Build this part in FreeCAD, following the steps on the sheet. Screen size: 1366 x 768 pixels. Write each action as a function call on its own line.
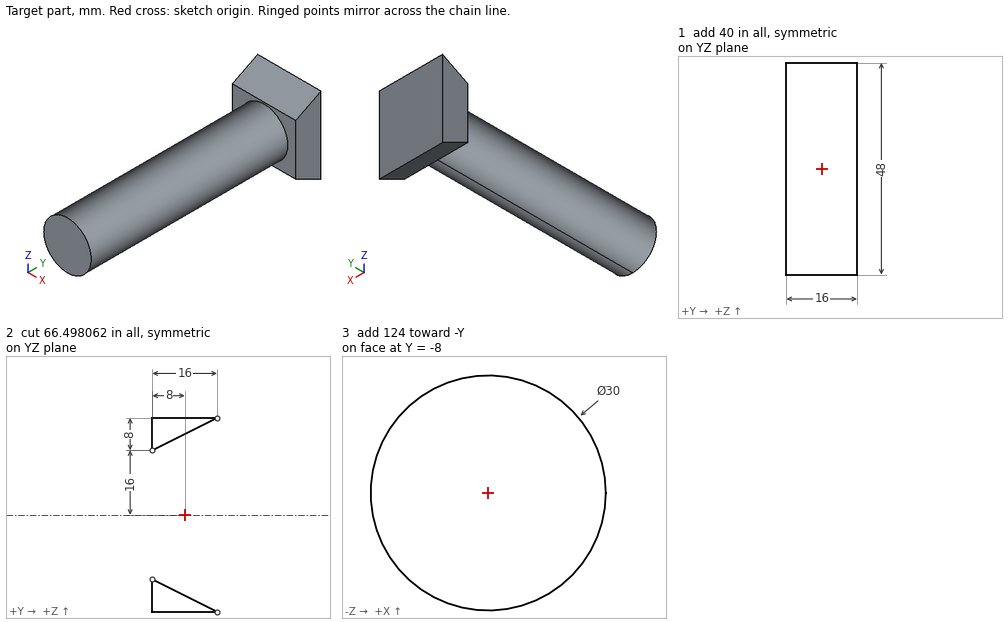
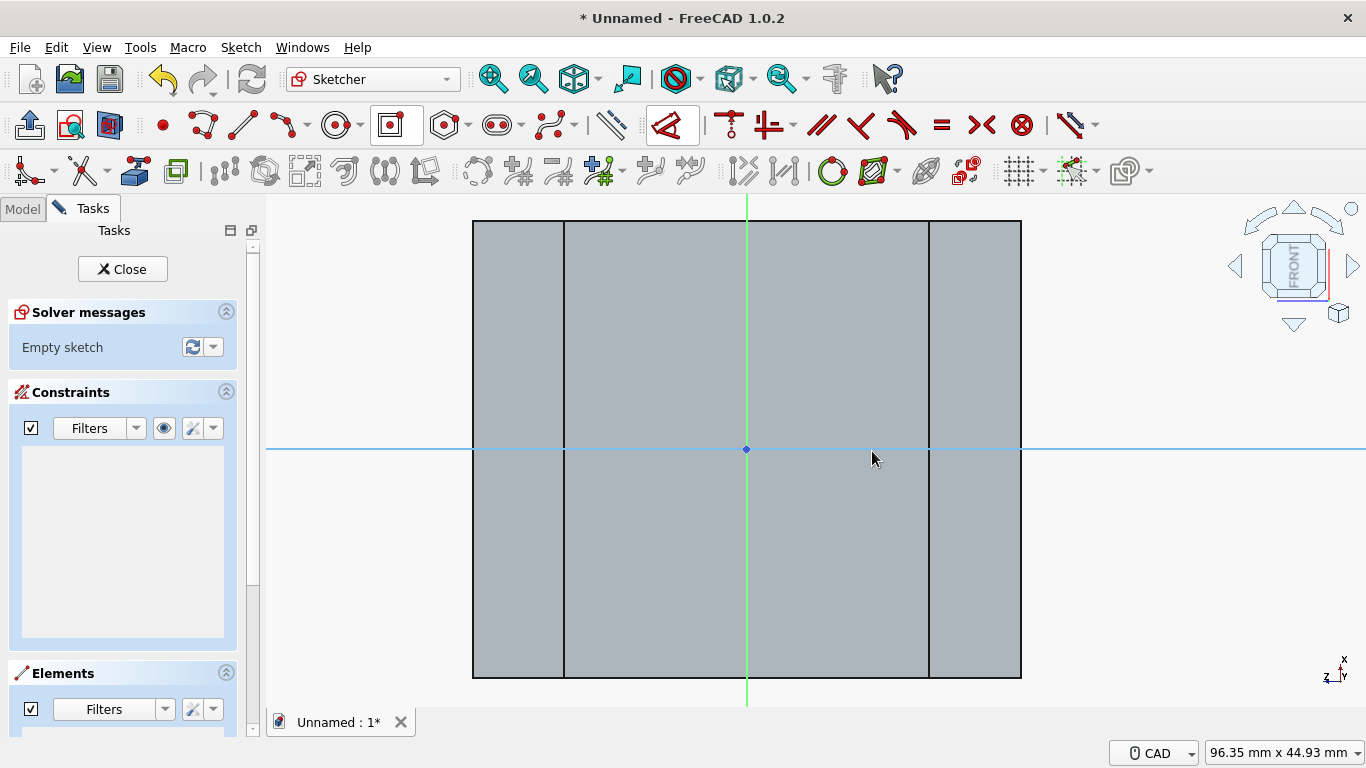
click(336, 126)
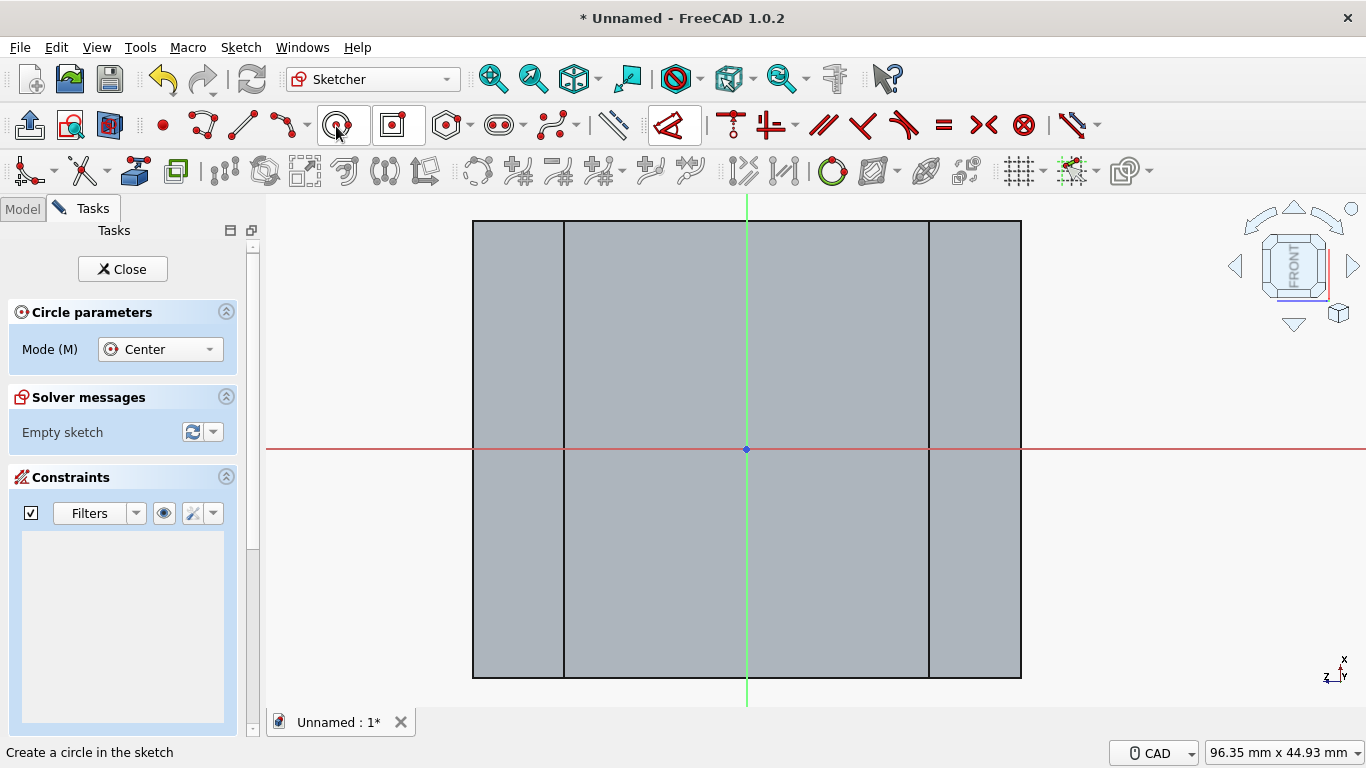
click(747, 449)
move(868, 328)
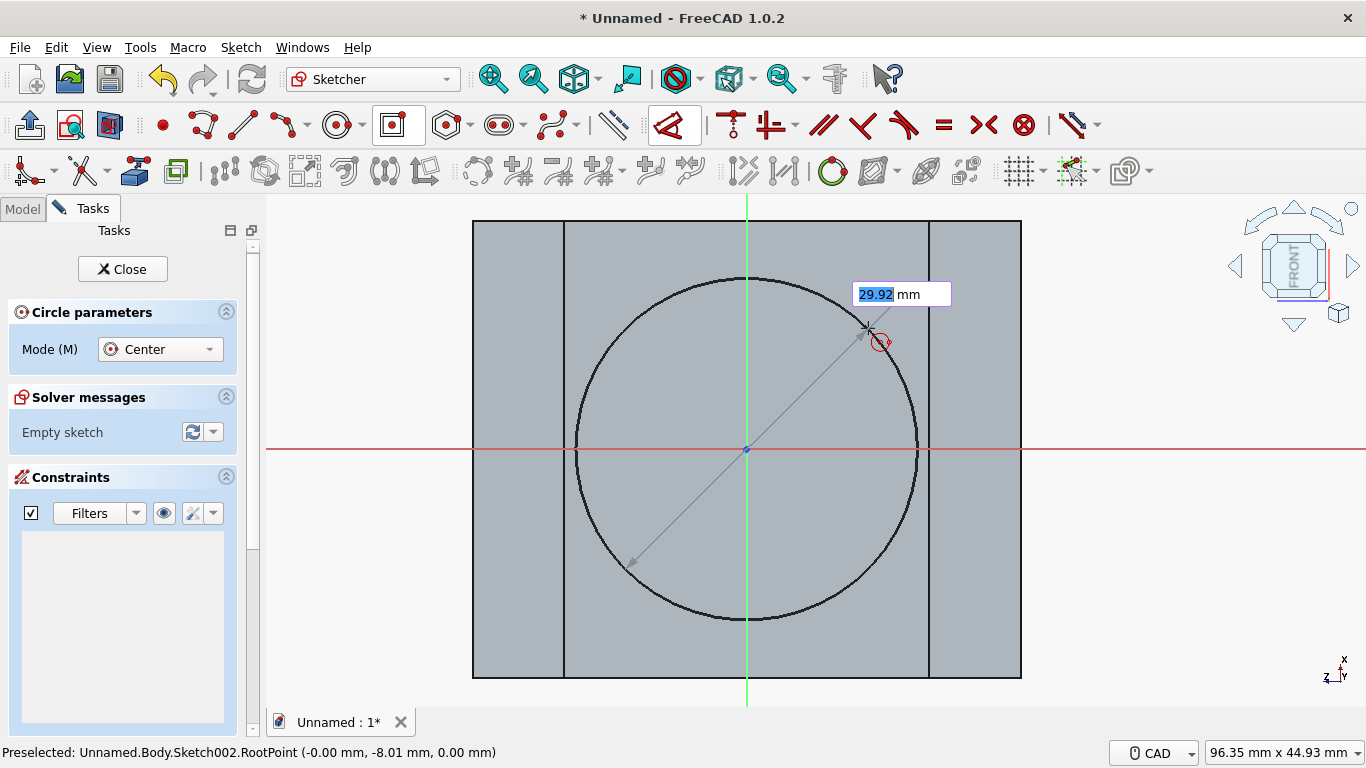
text(30)
key(Return)
key(Escape)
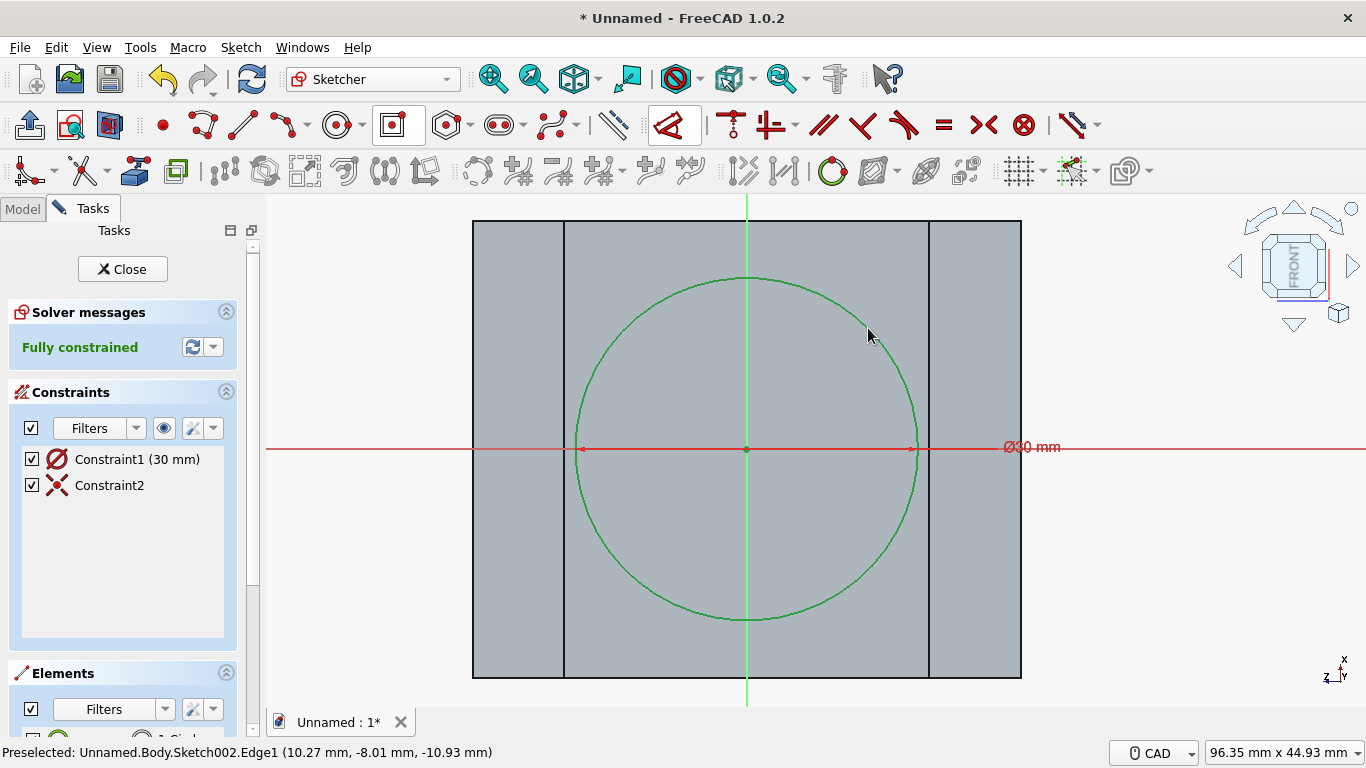
click(123, 269)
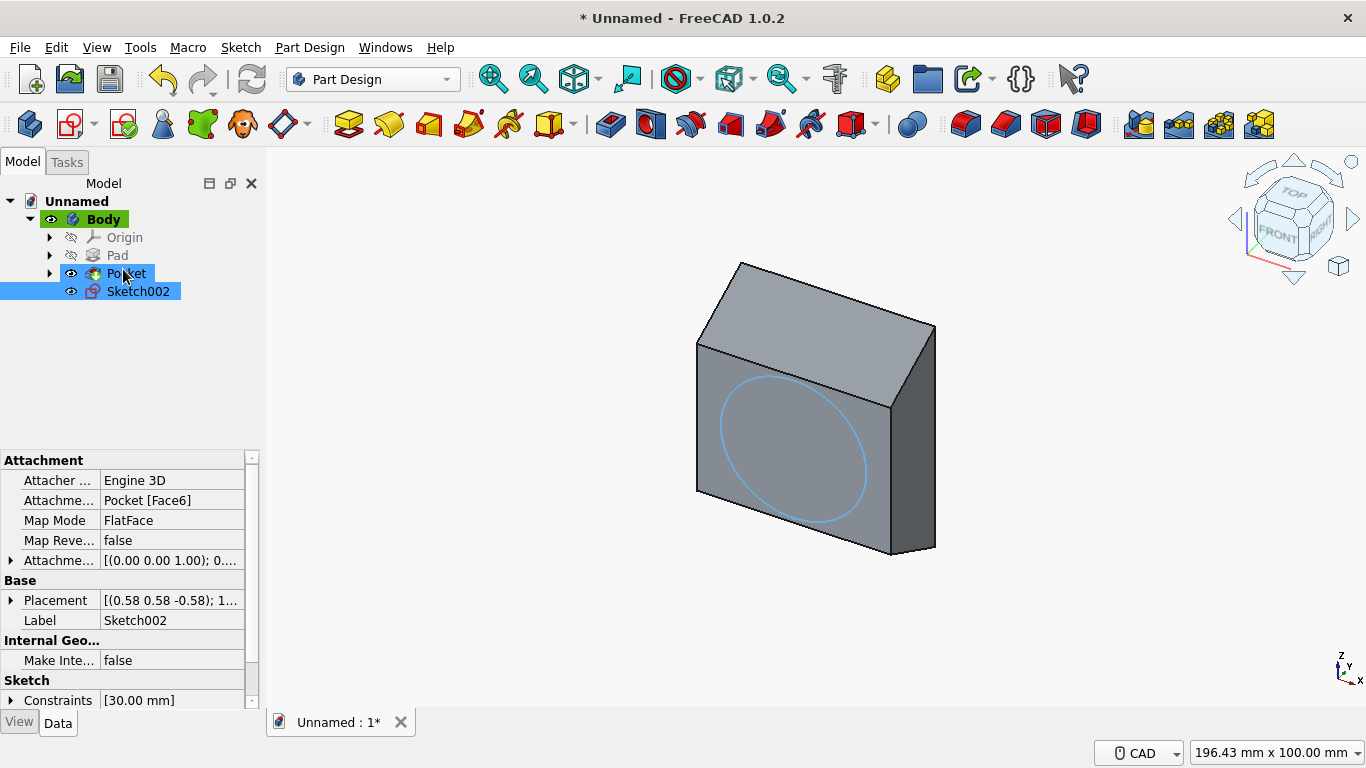
click(350, 124)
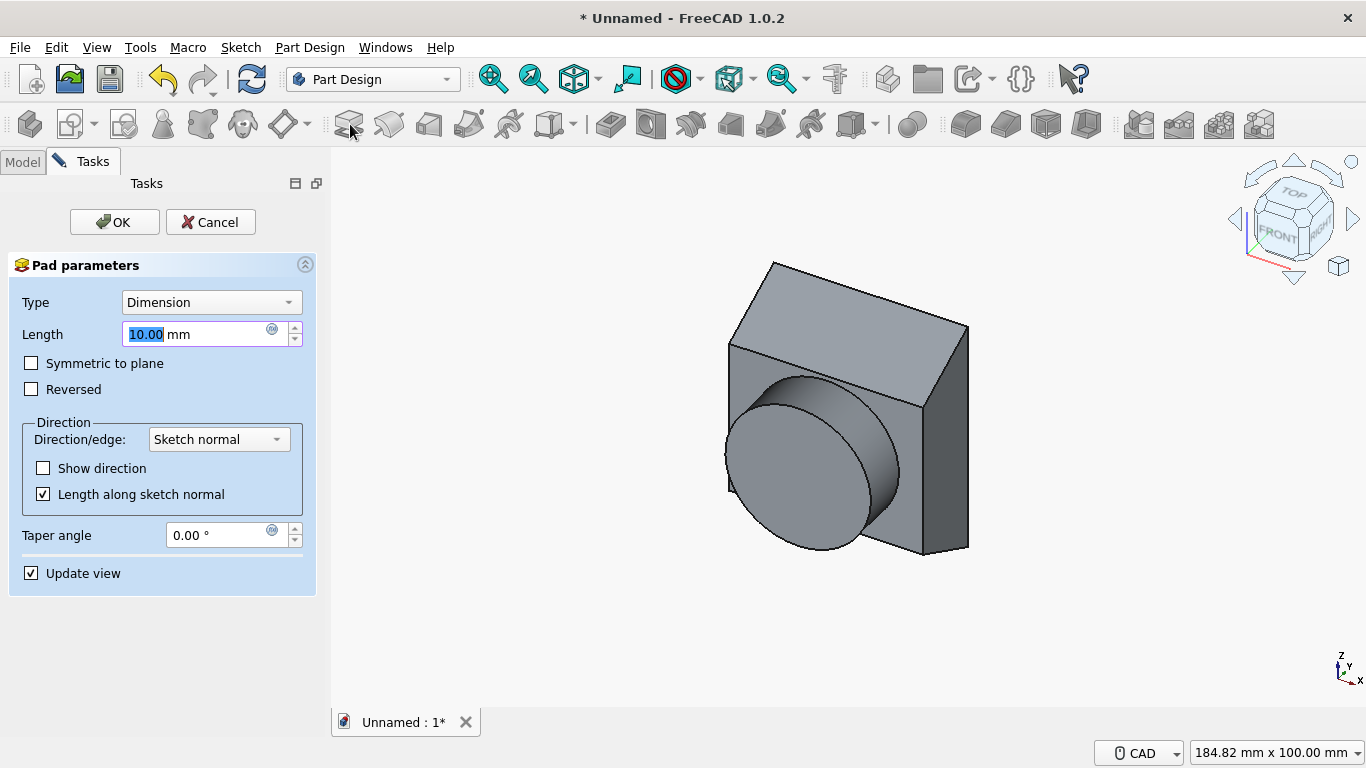
text(124)
key(Tab)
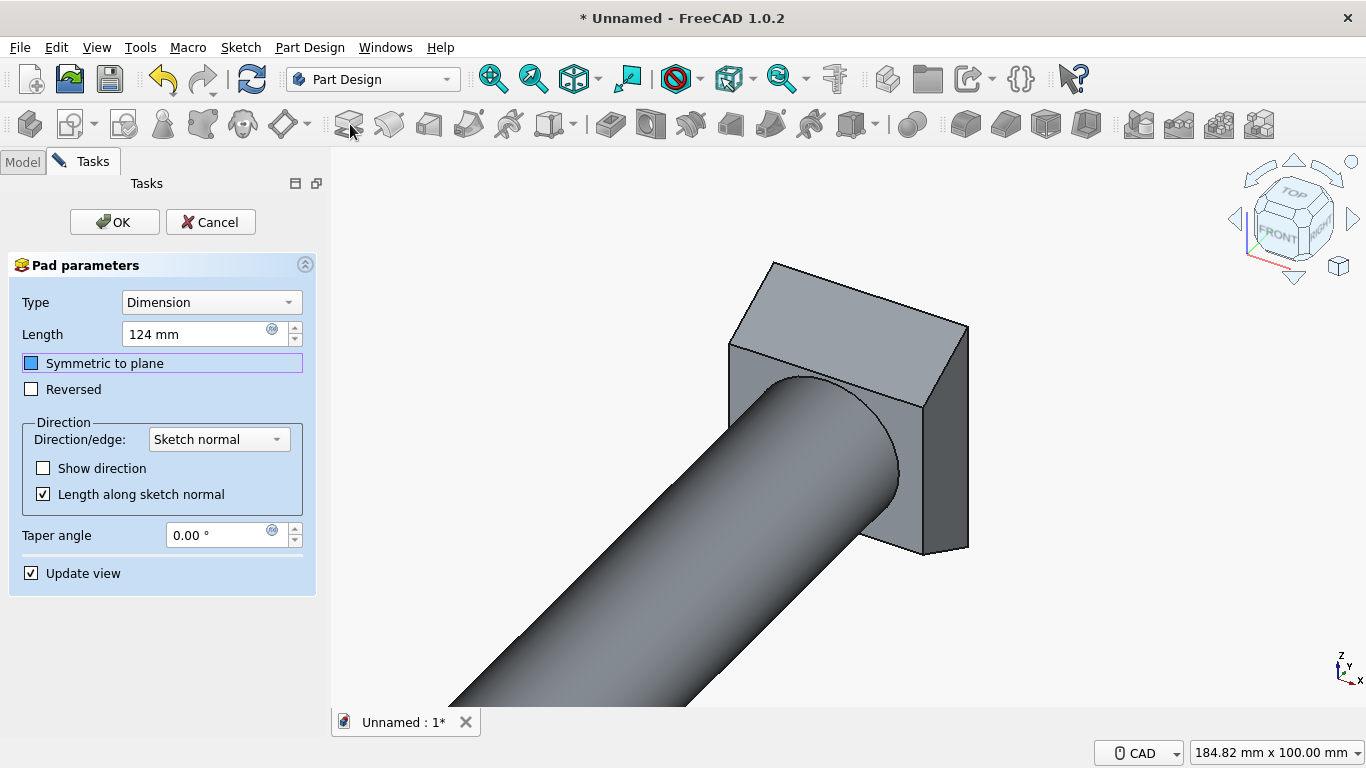
click(115, 222)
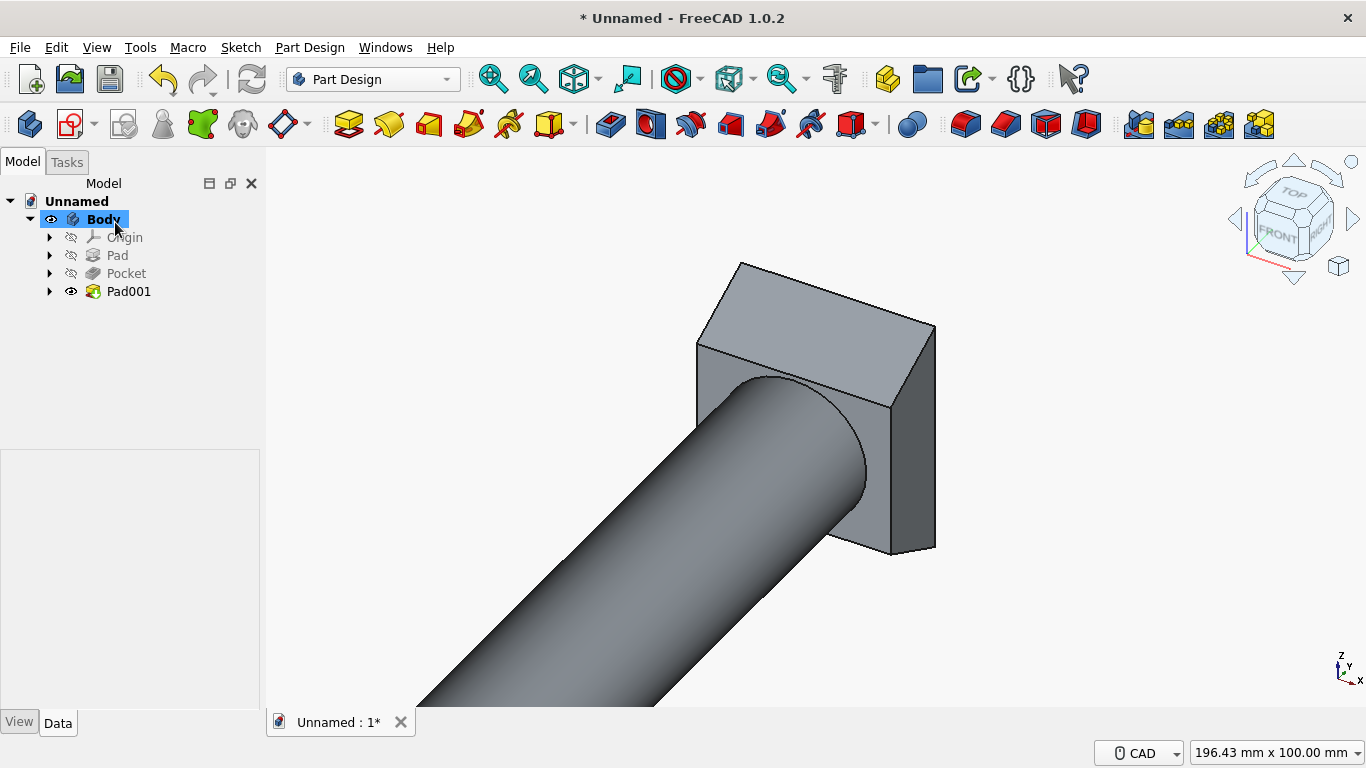
key(0)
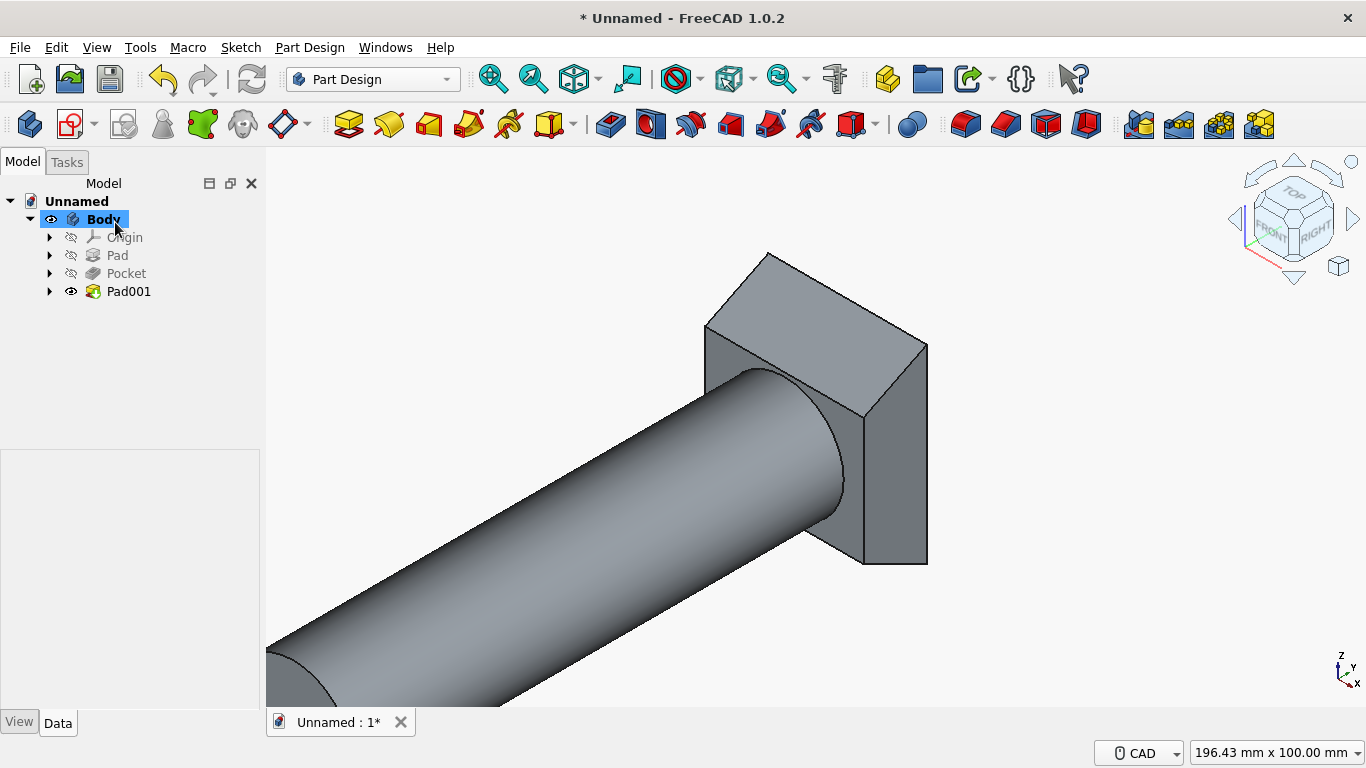
key(v)
key(f)